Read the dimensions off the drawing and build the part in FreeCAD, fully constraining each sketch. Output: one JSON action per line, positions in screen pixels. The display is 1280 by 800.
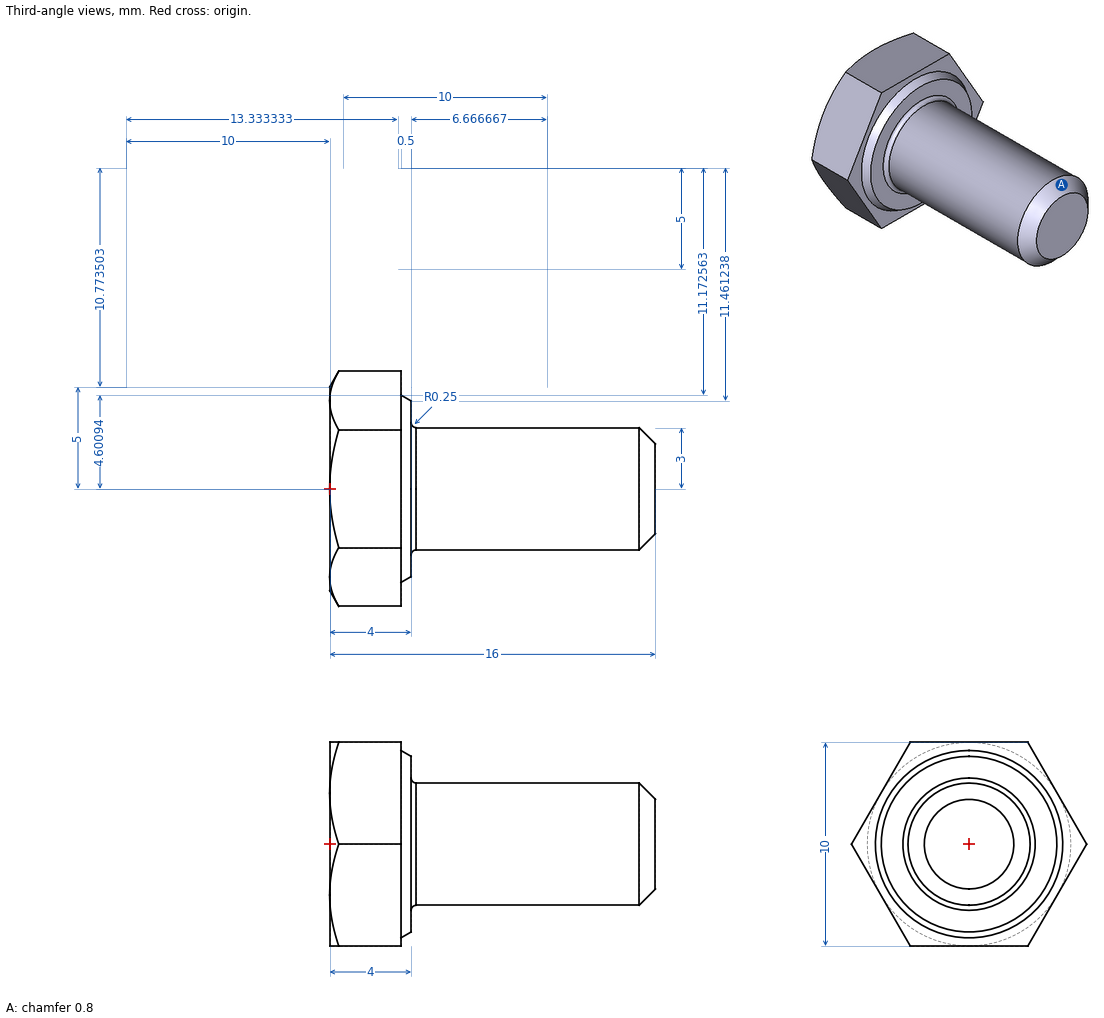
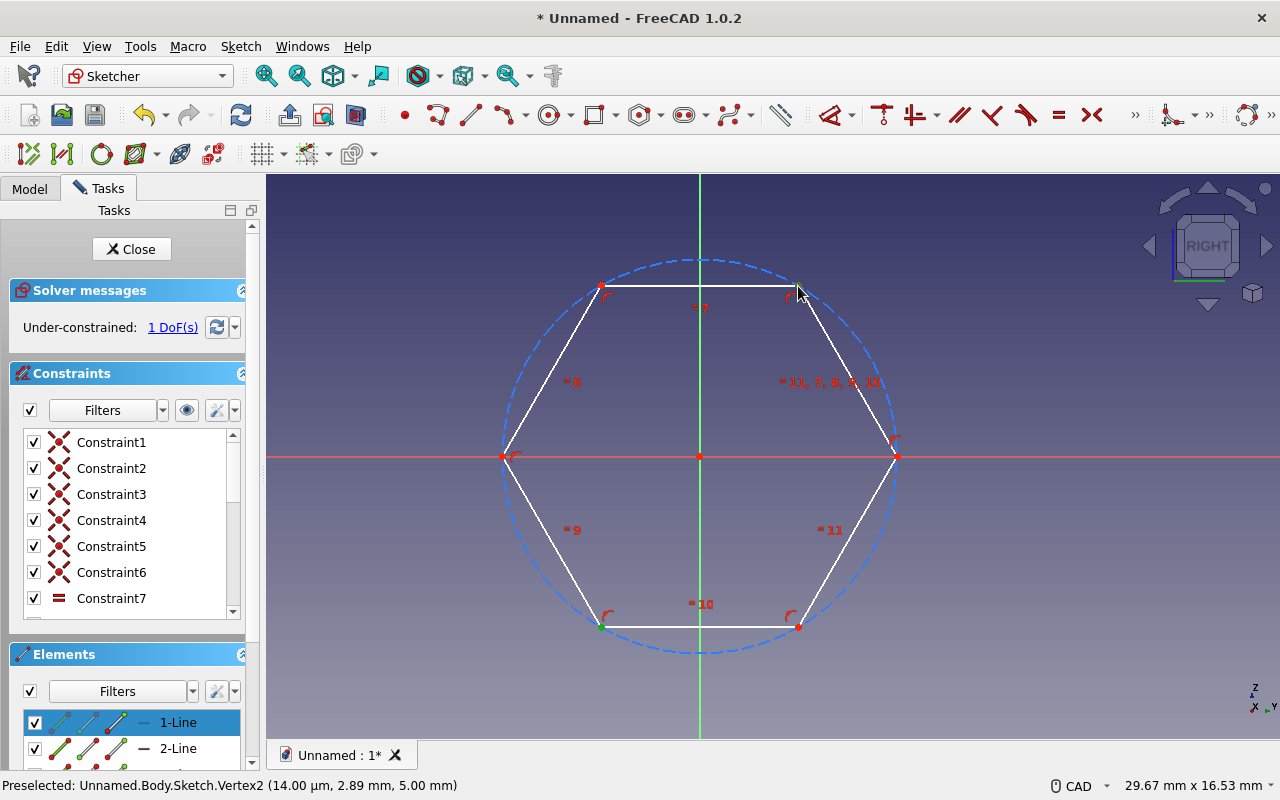
{"action": "key", "text": "i"}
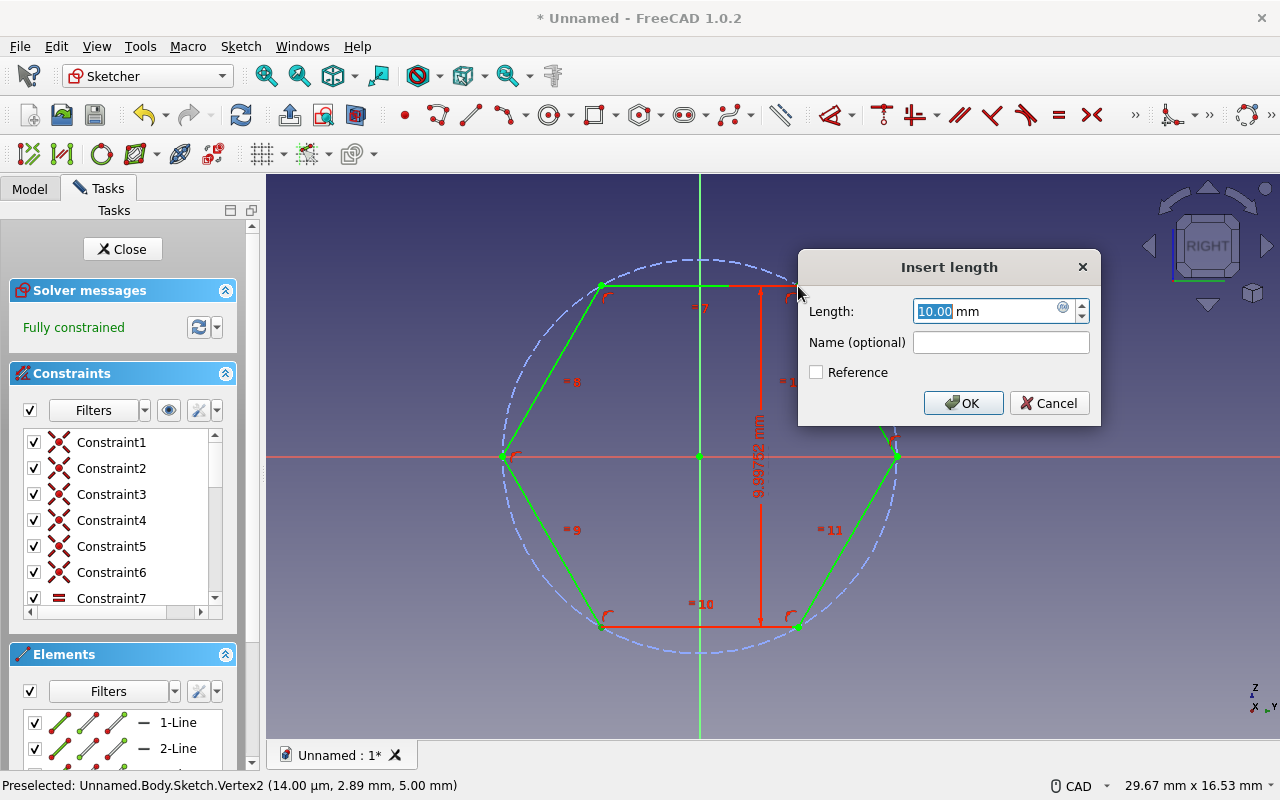
{"action": "type", "text": "10"}
{"action": "key", "text": "Return"}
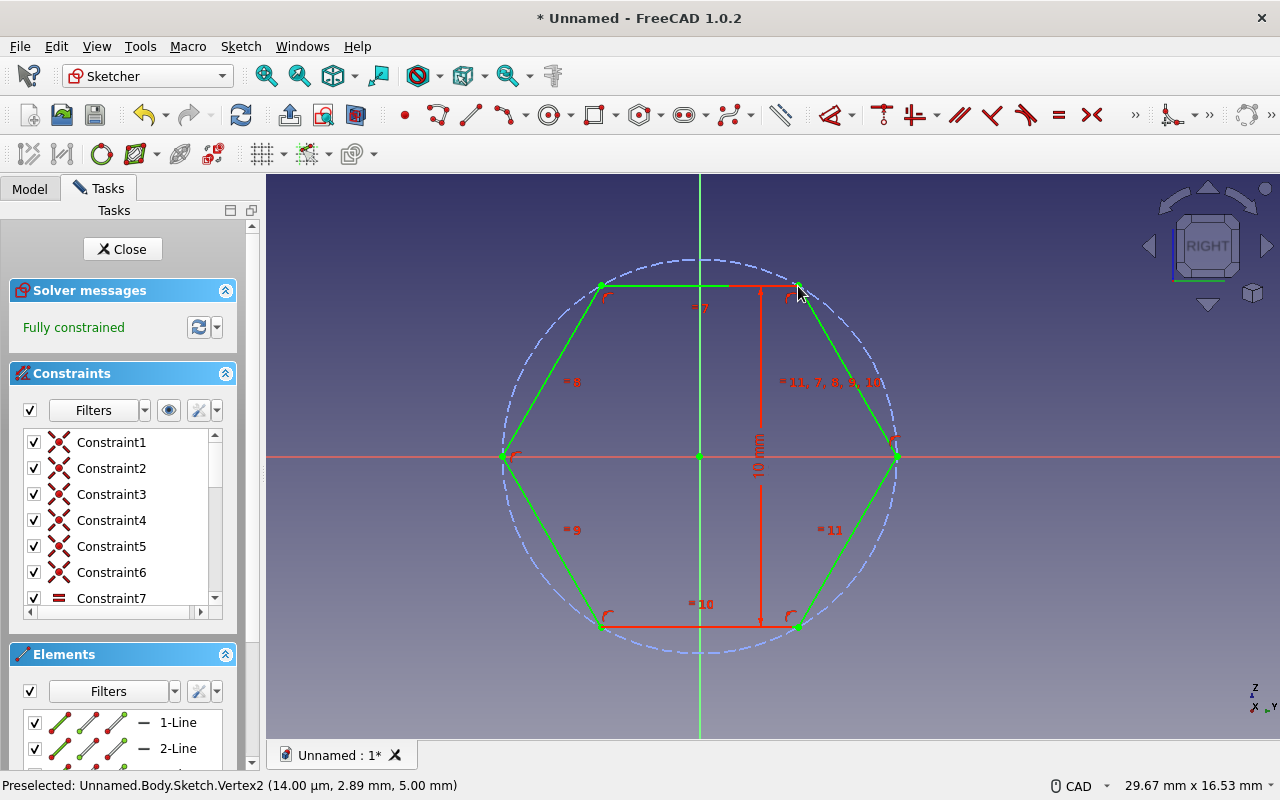
{"action": "left_click", "coordinate": [123, 249]}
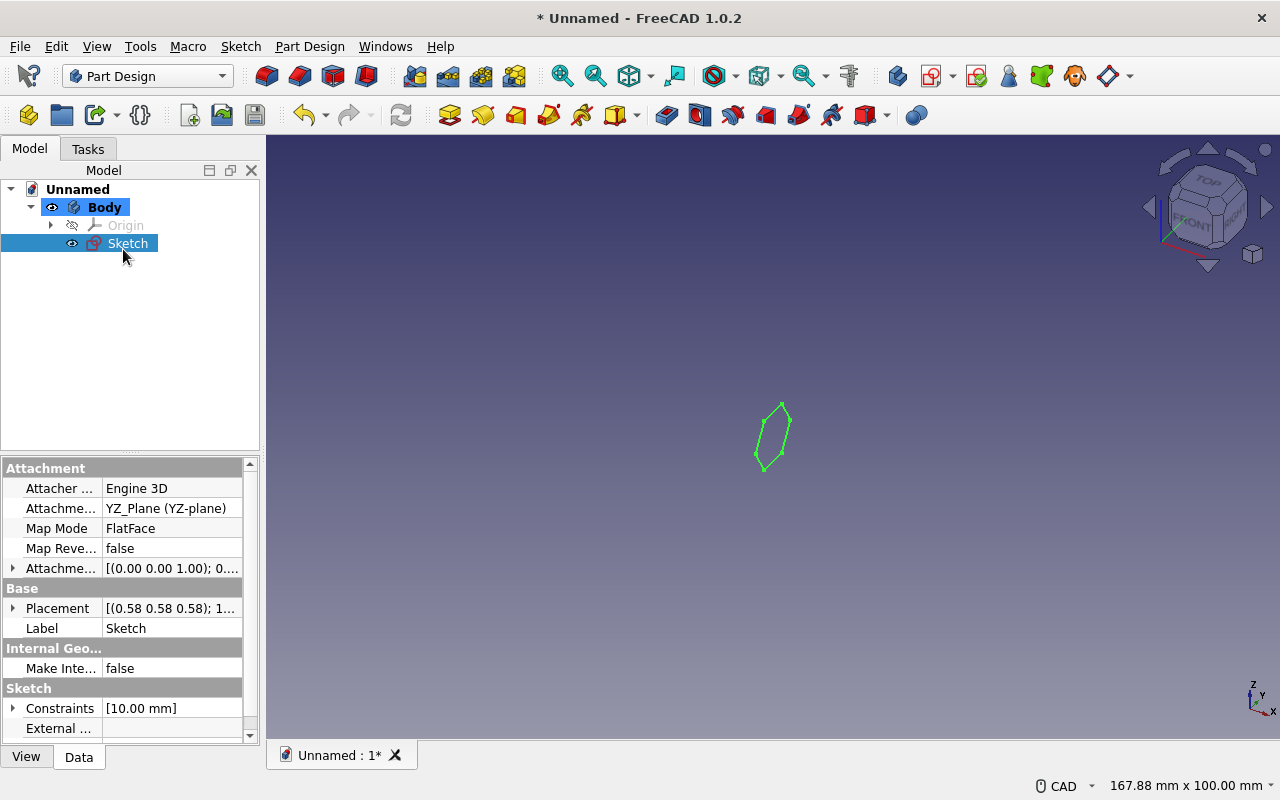
{"action": "left_click", "coordinate": [450, 116]}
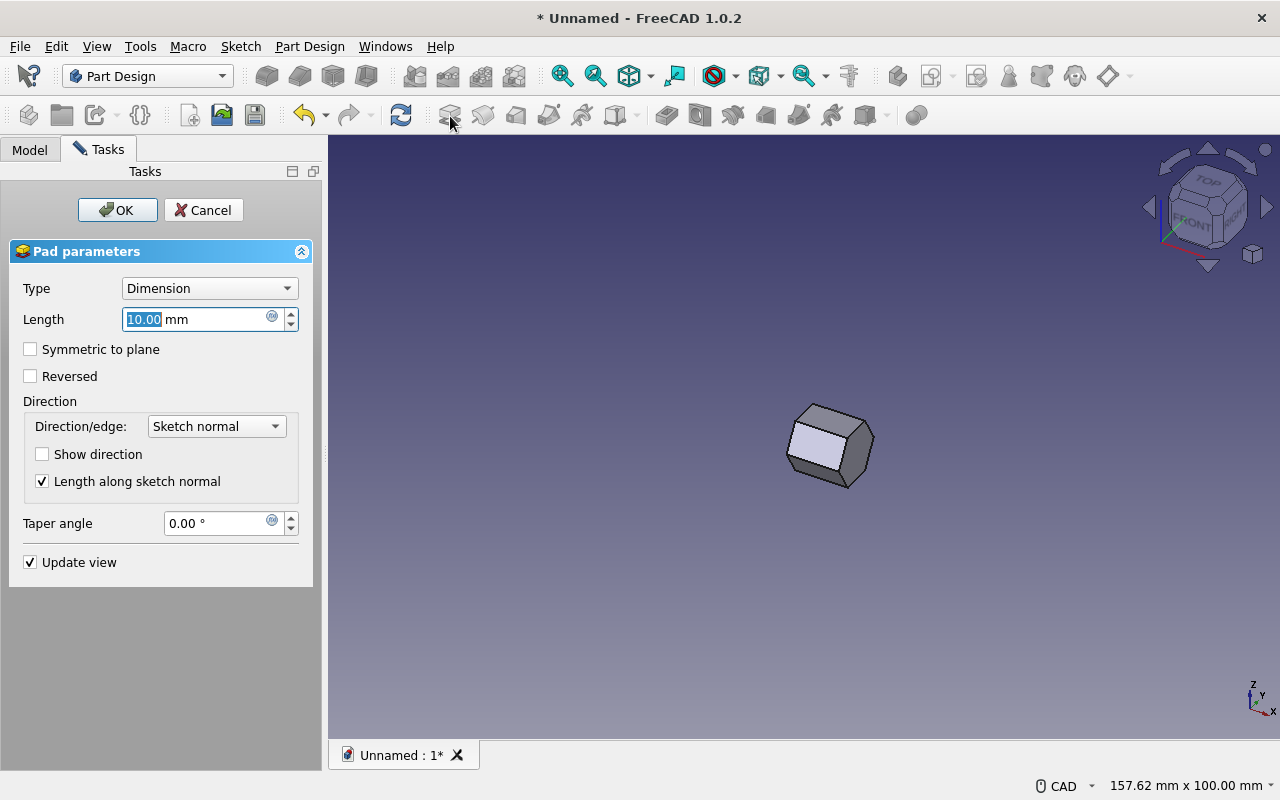
{"action": "type", "text": "4"}
{"action": "key", "text": "Tab"}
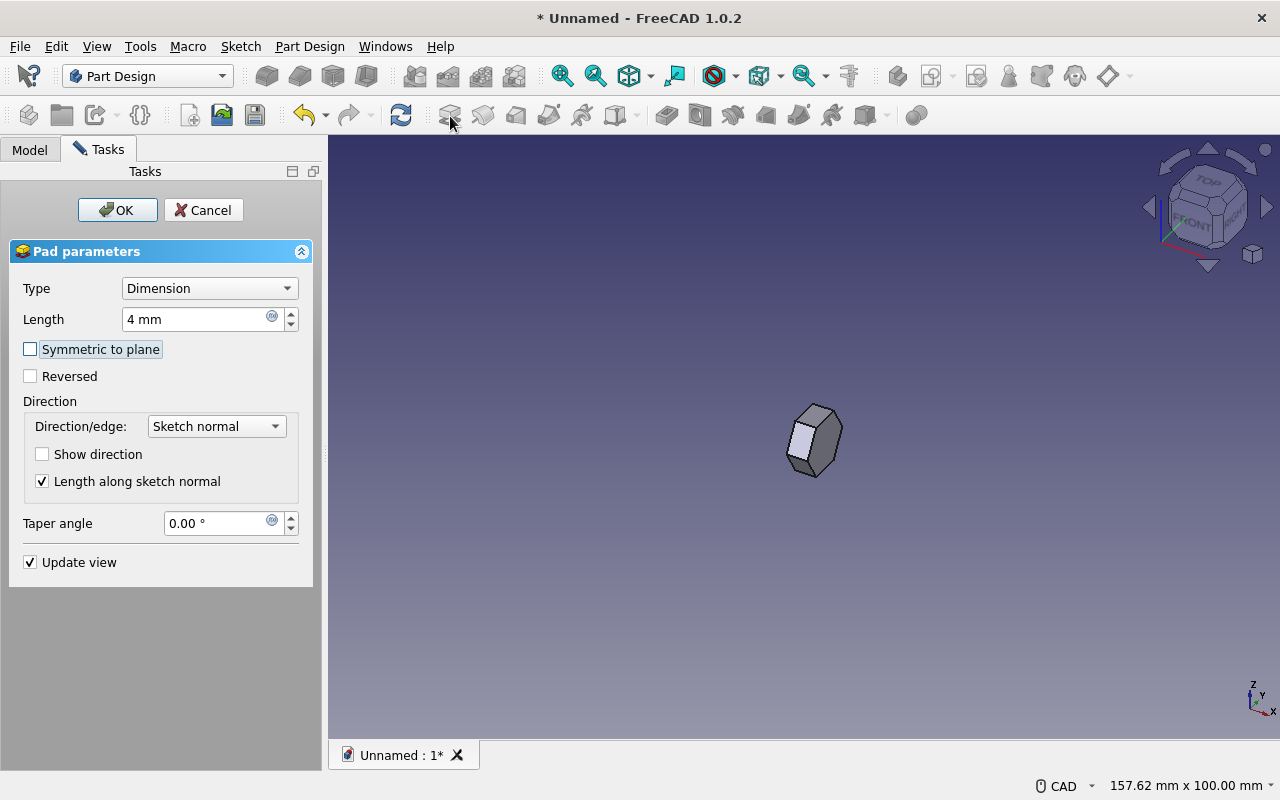
{"action": "left_click", "coordinate": [118, 210]}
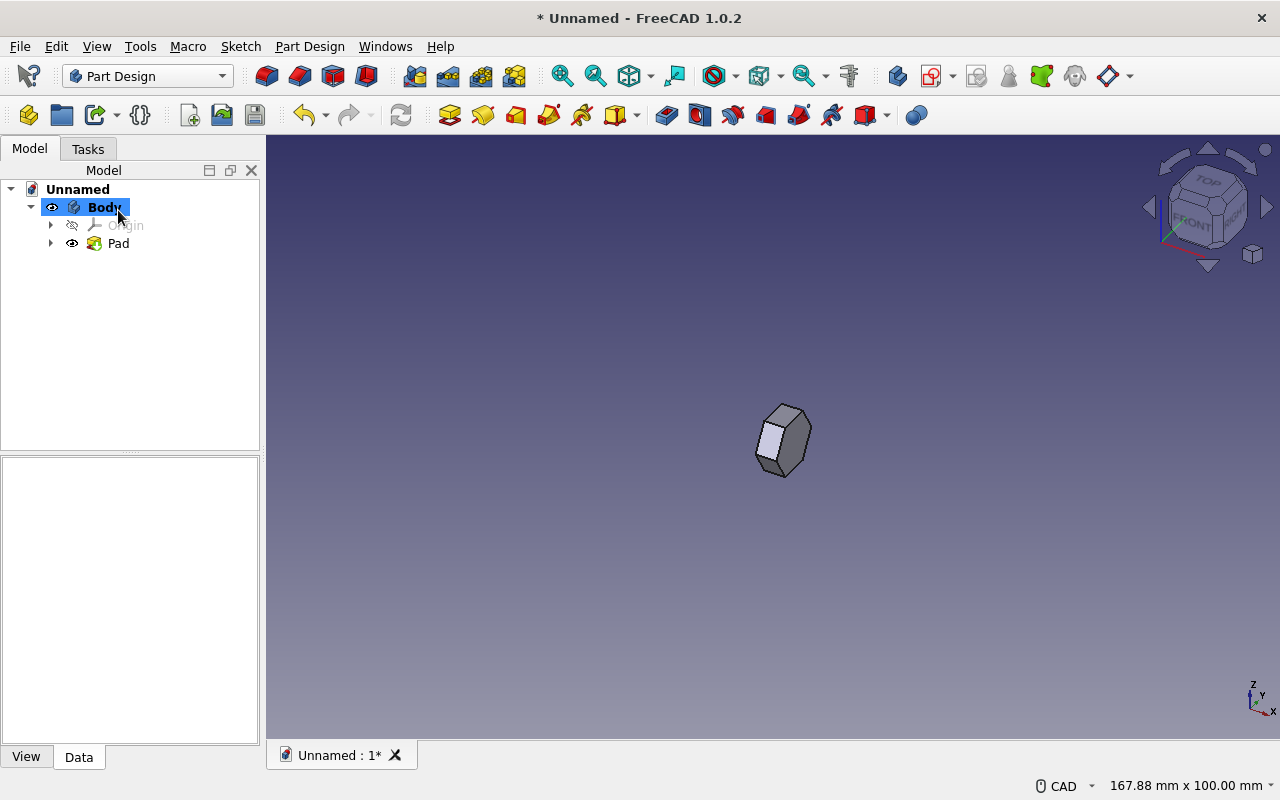
{"action": "left_click", "coordinate": [563, 76]}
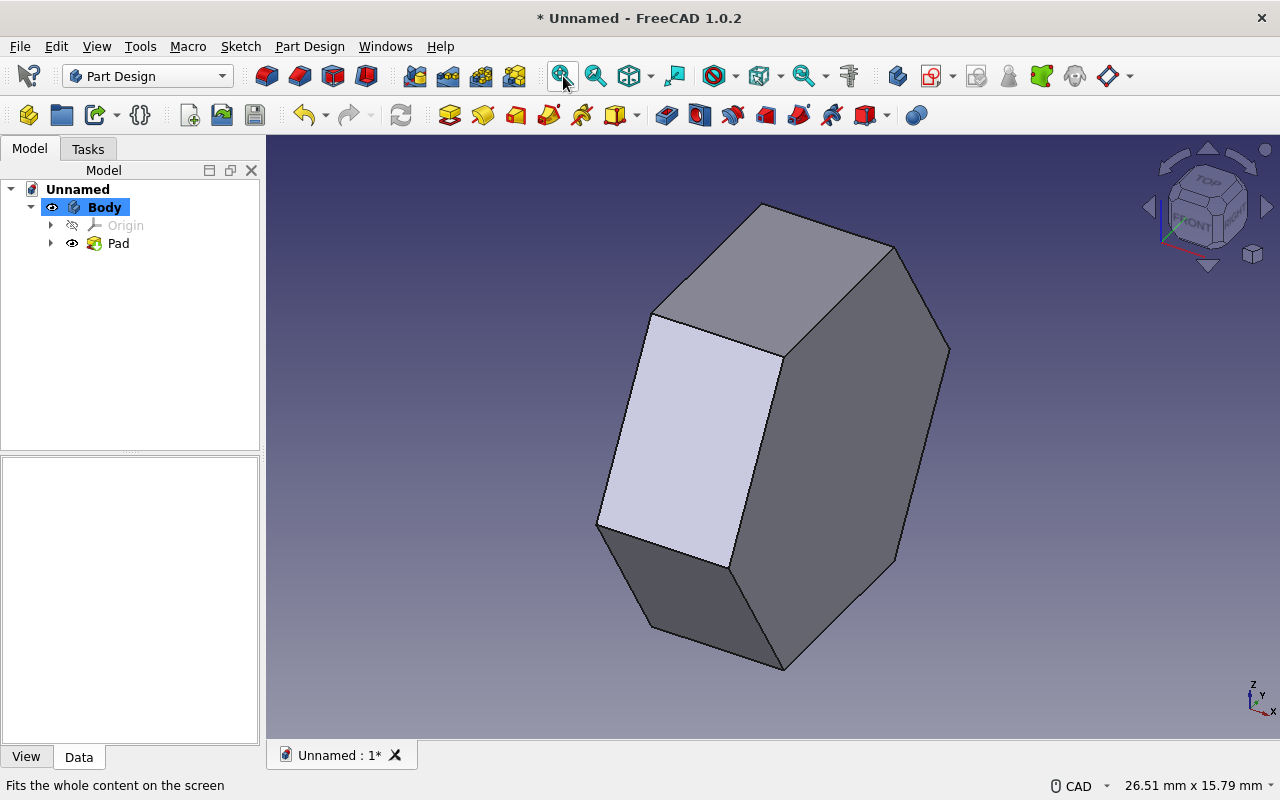
{"action": "left_click", "coordinate": [930, 76]}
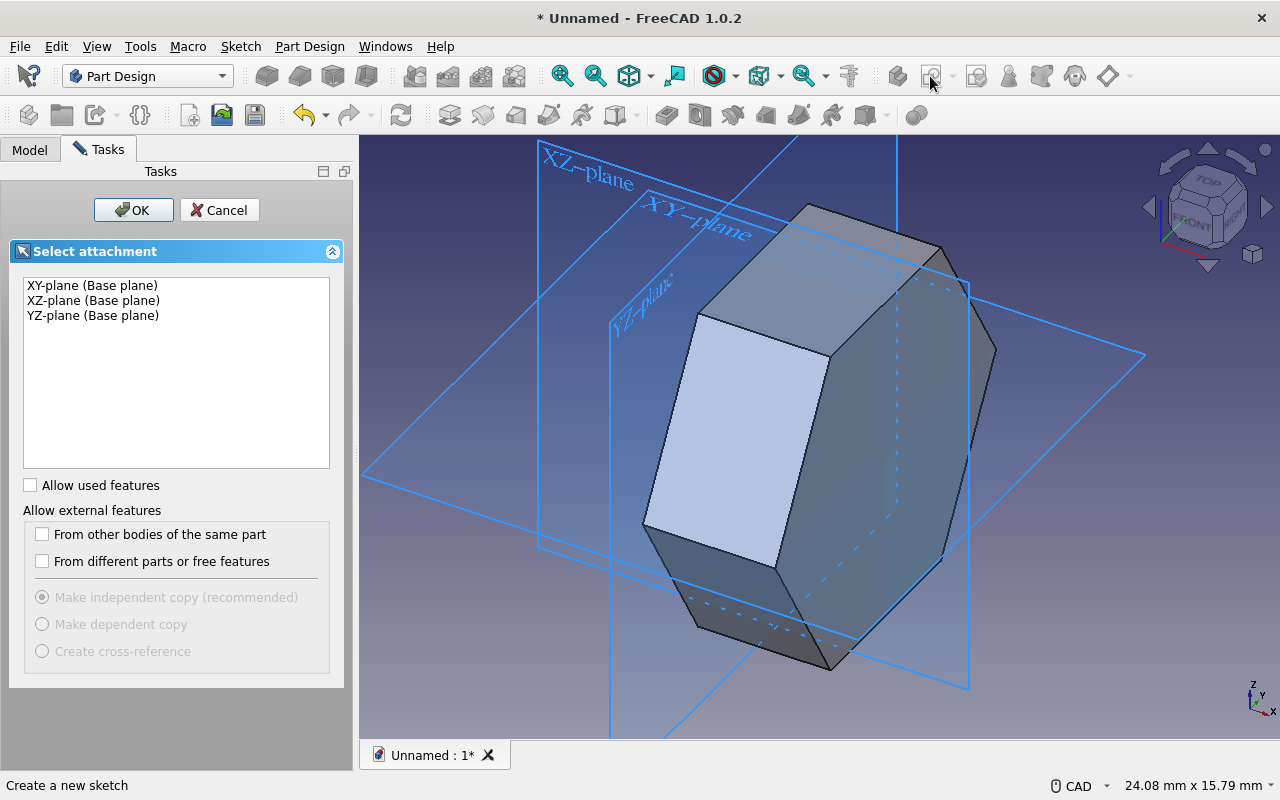
{"action": "left_click", "coordinate": [84, 286]}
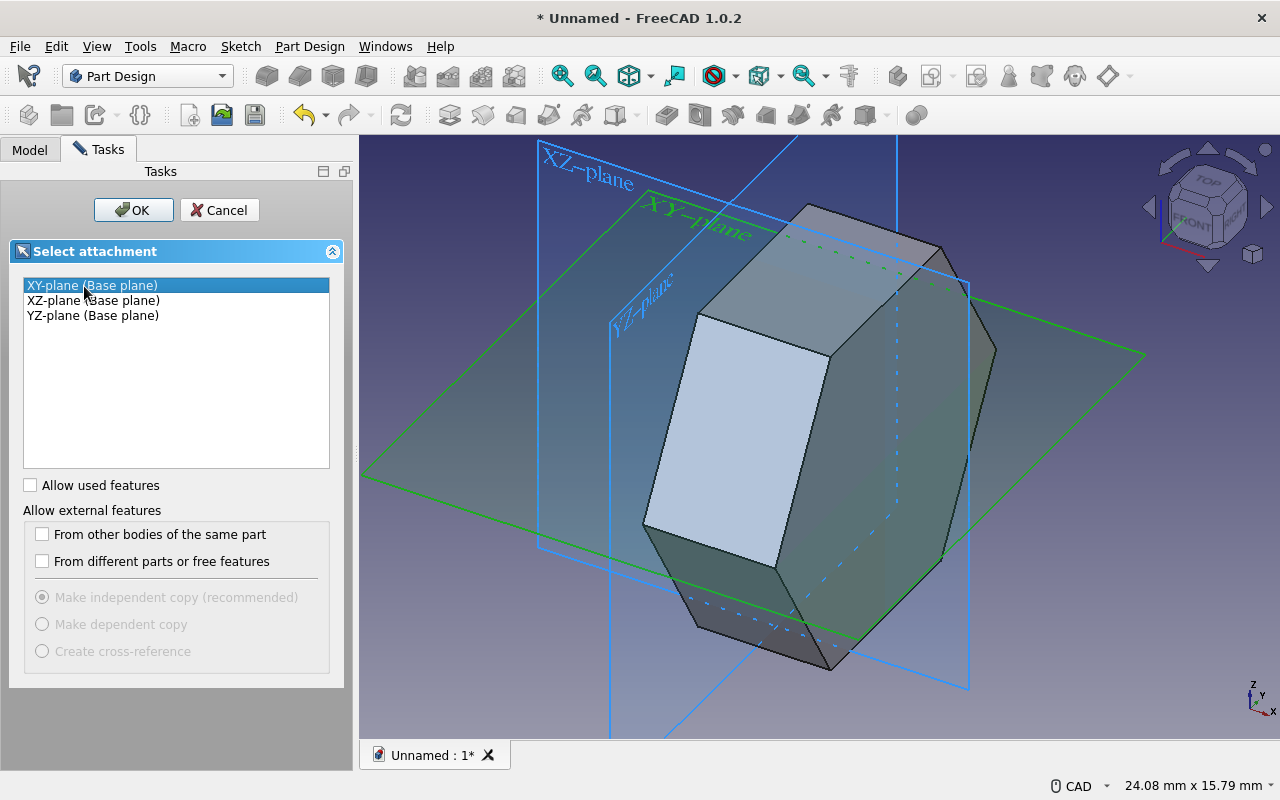
{"action": "left_click", "coordinate": [134, 210]}